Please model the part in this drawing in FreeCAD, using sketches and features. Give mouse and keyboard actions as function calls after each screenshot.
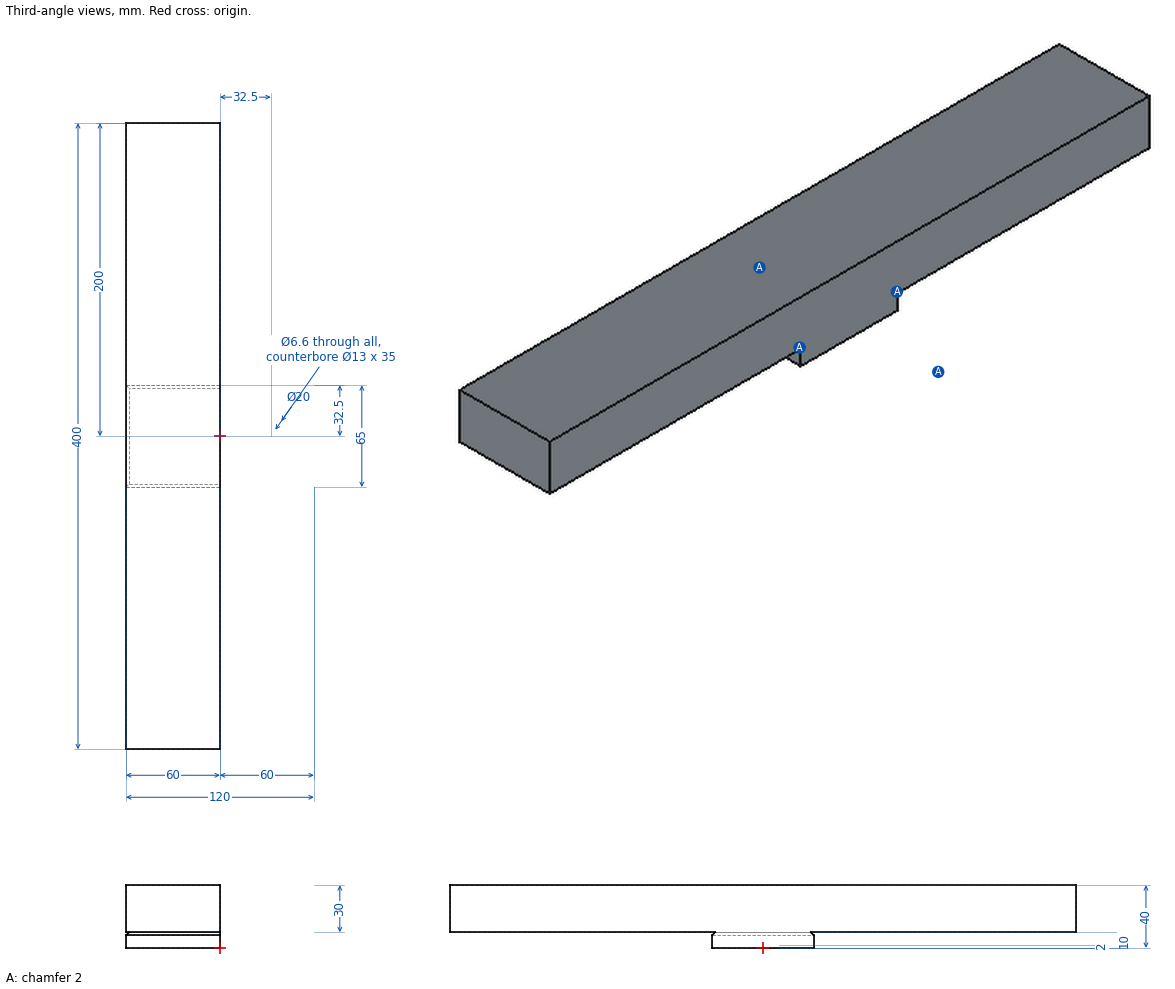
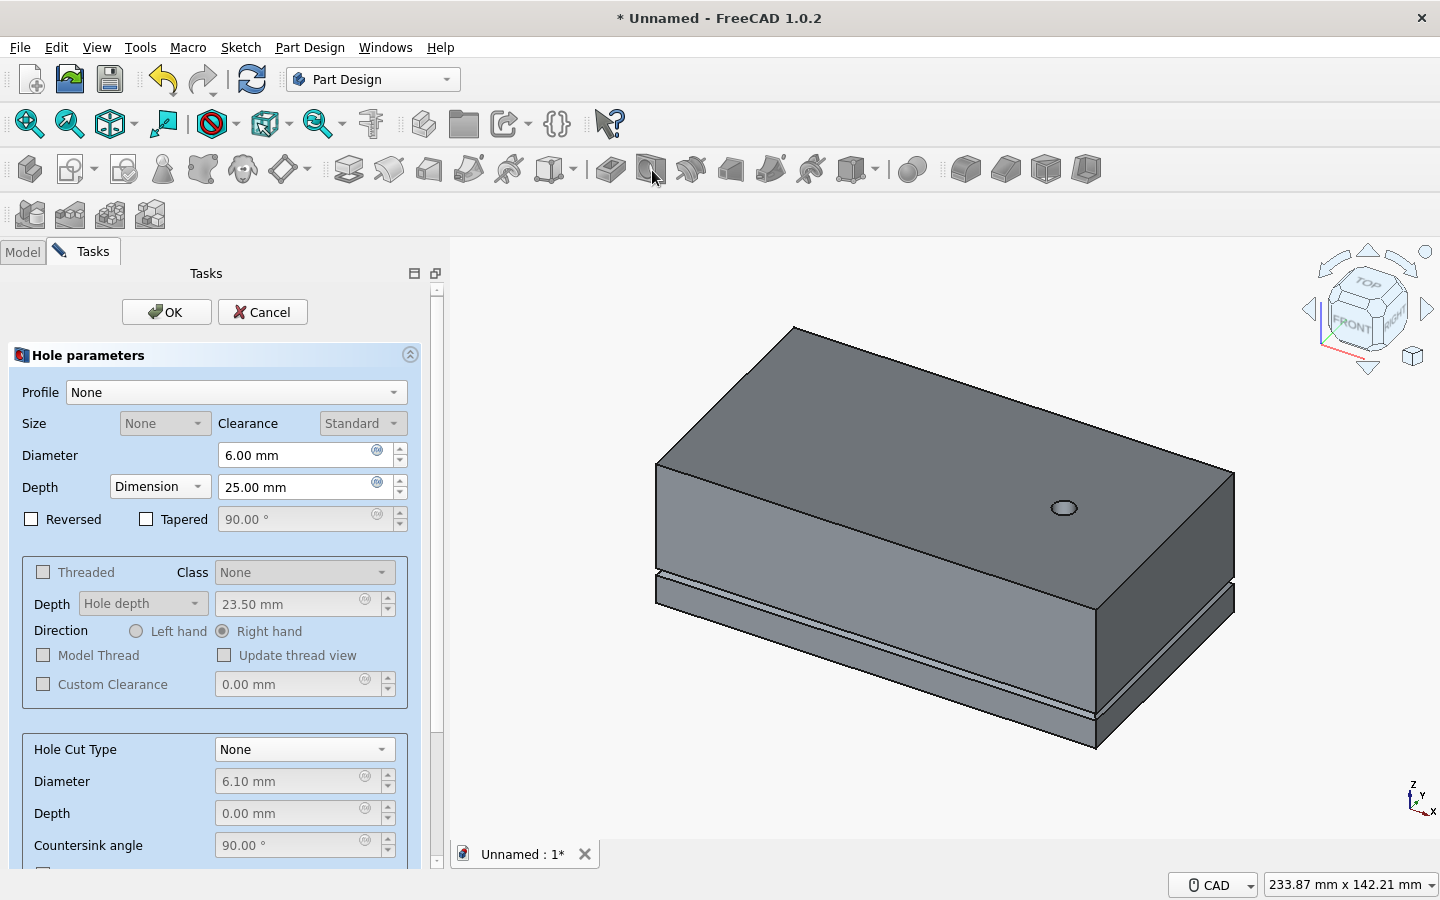
triple_click(305, 455)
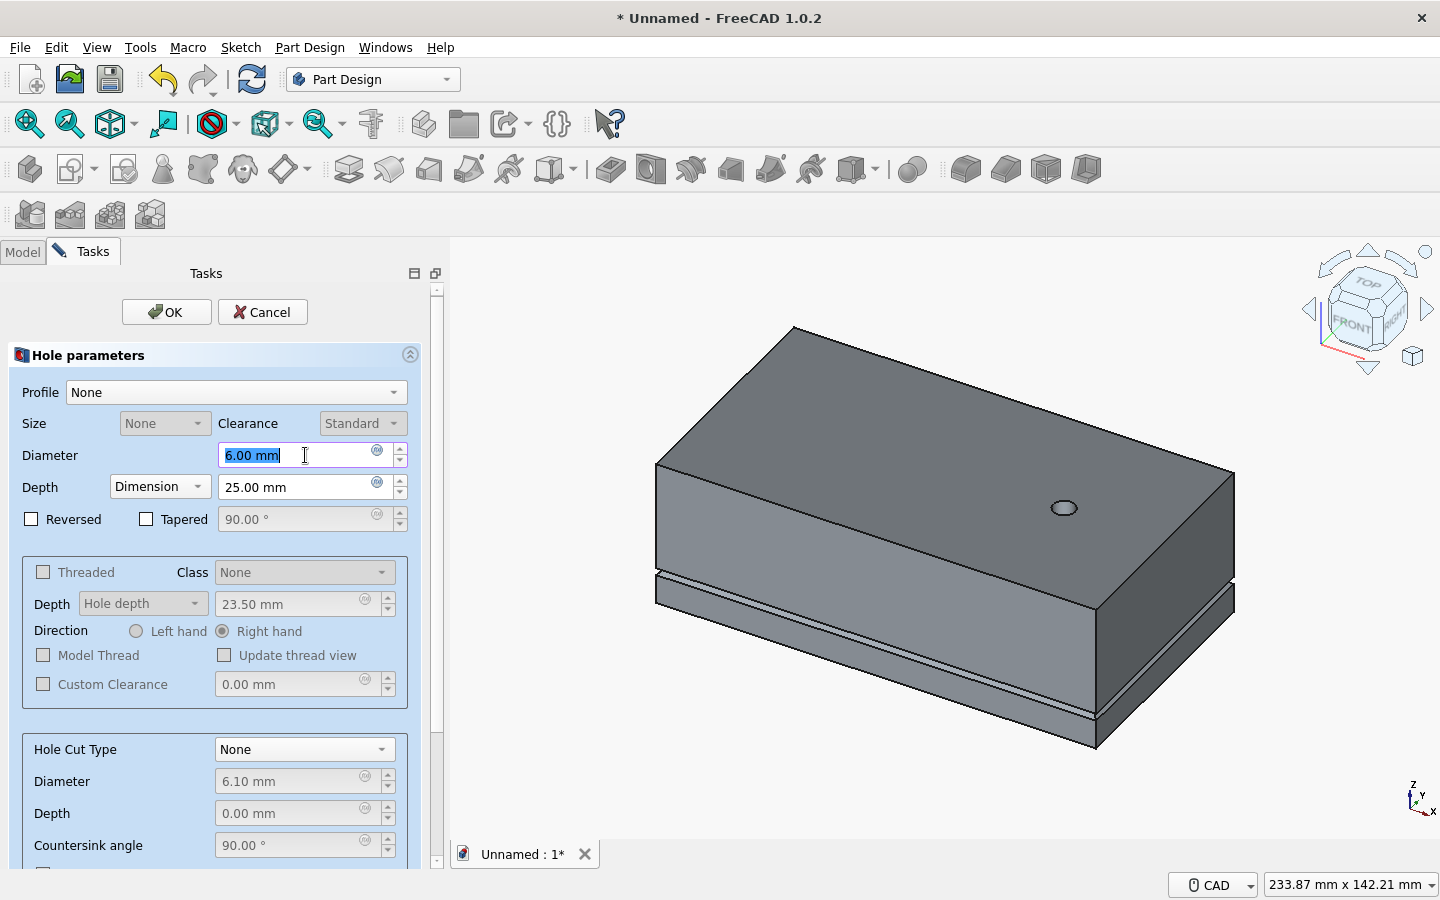
text(6.6)
key(Tab)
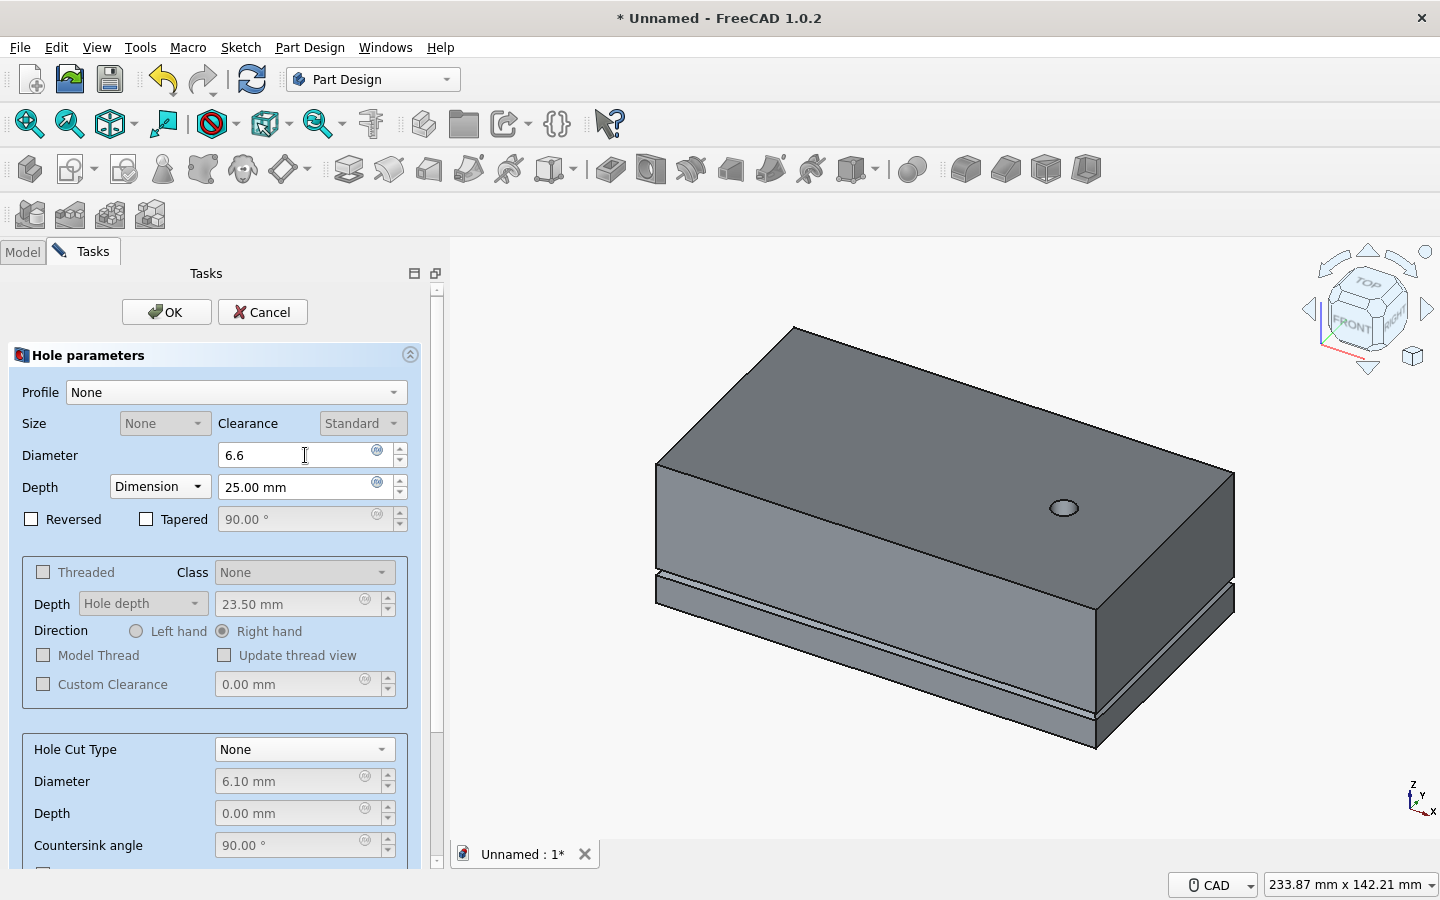
click(161, 486)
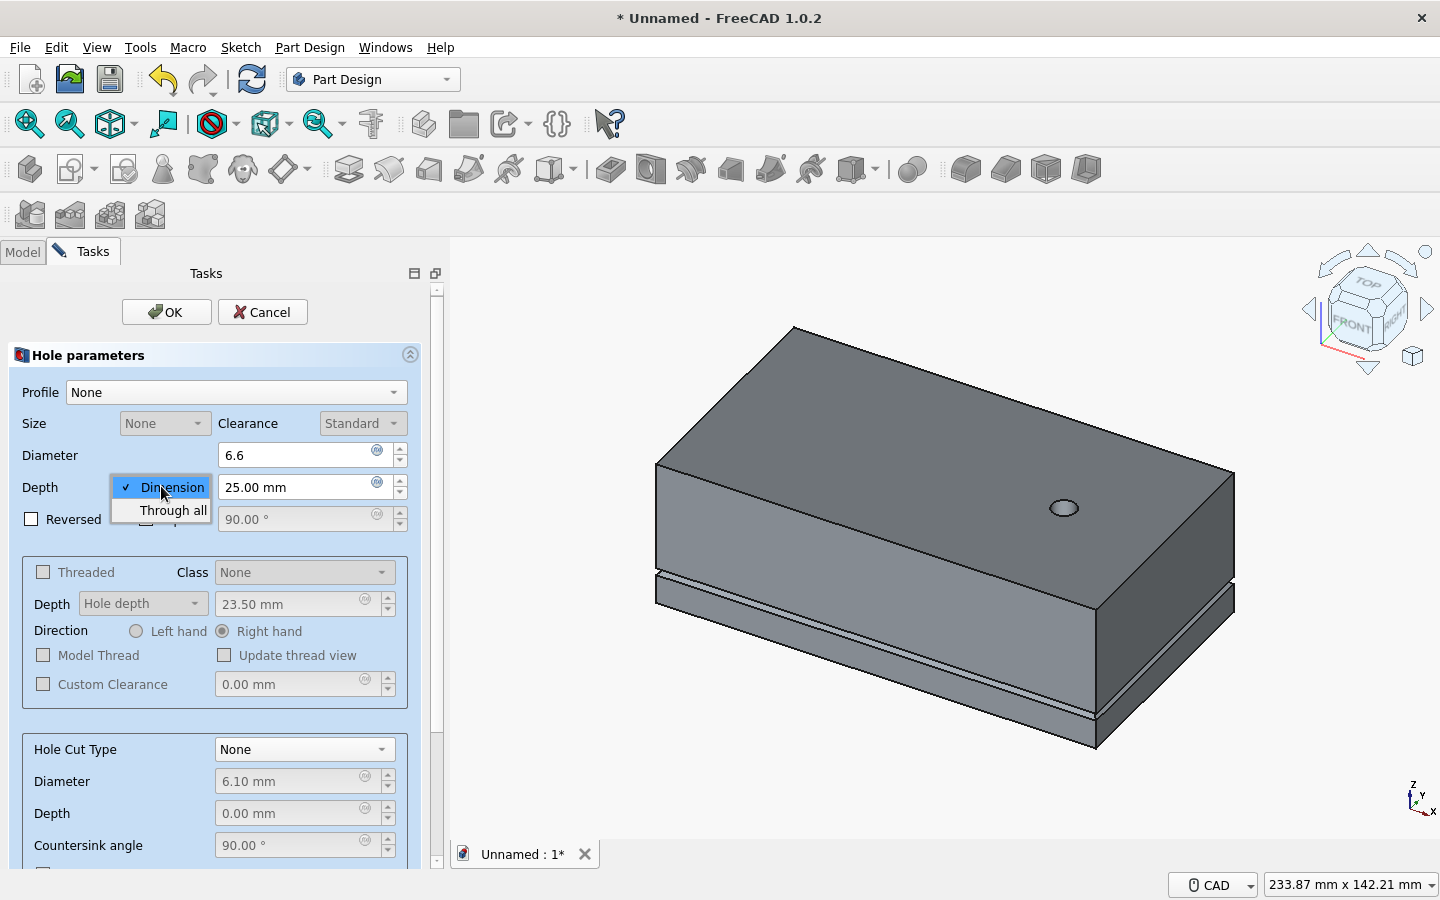
click(160, 510)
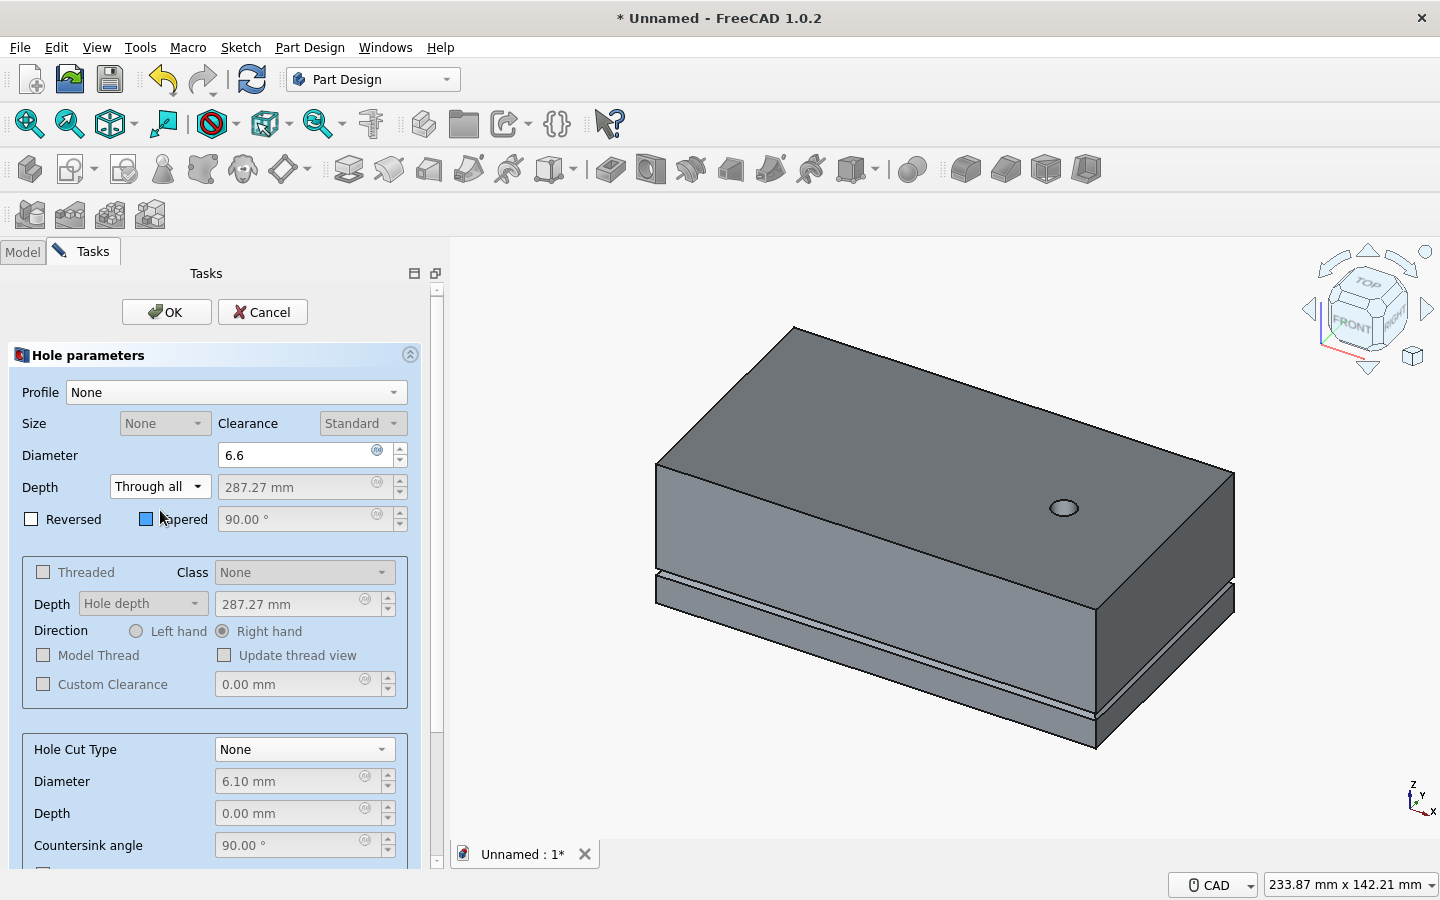
click(306, 750)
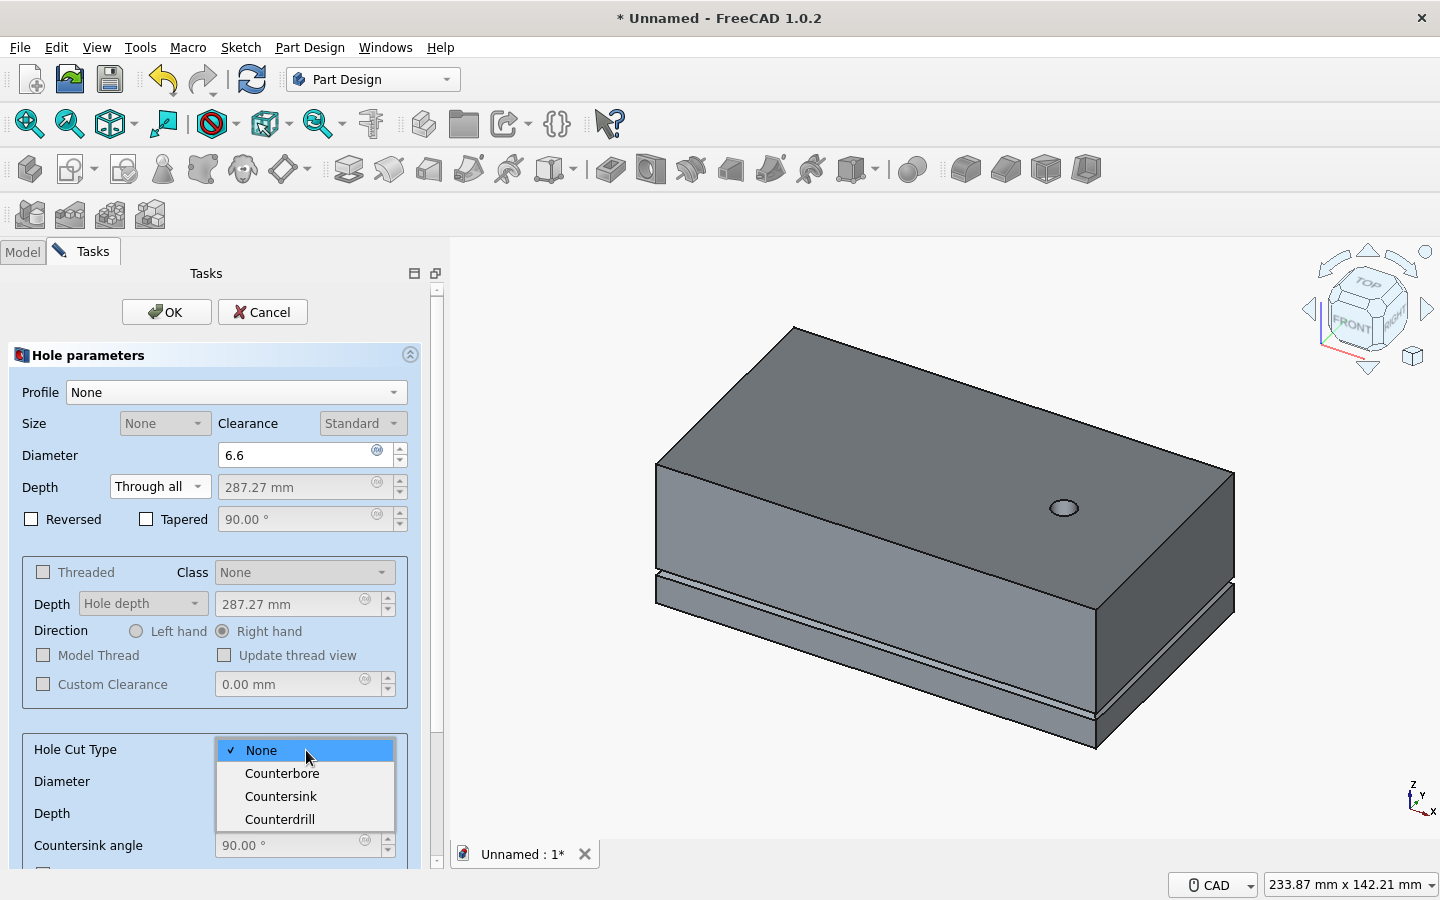
click(304, 774)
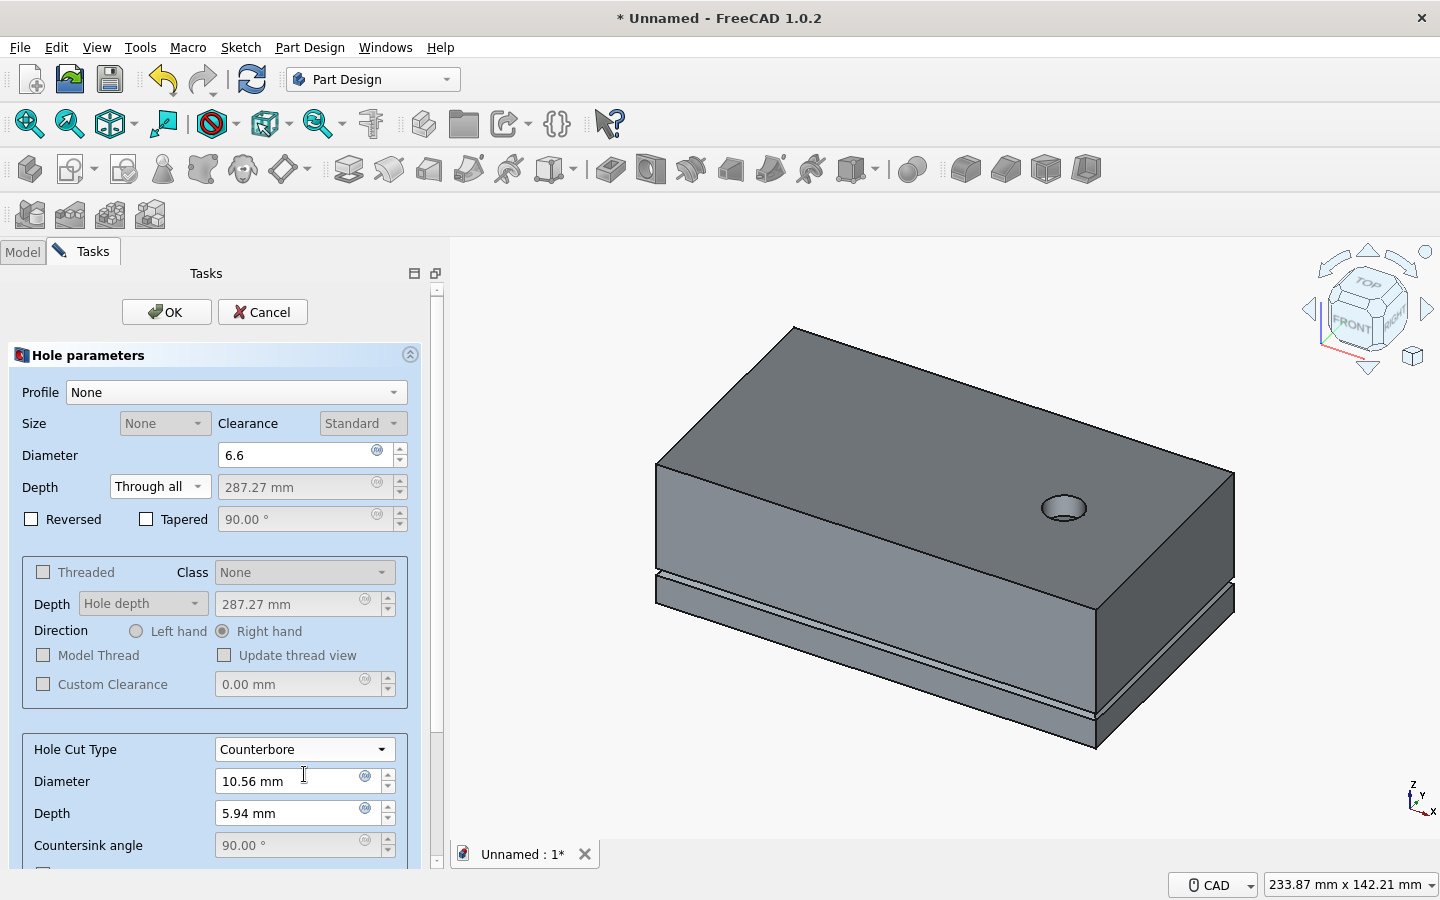
triple_click(298, 781)